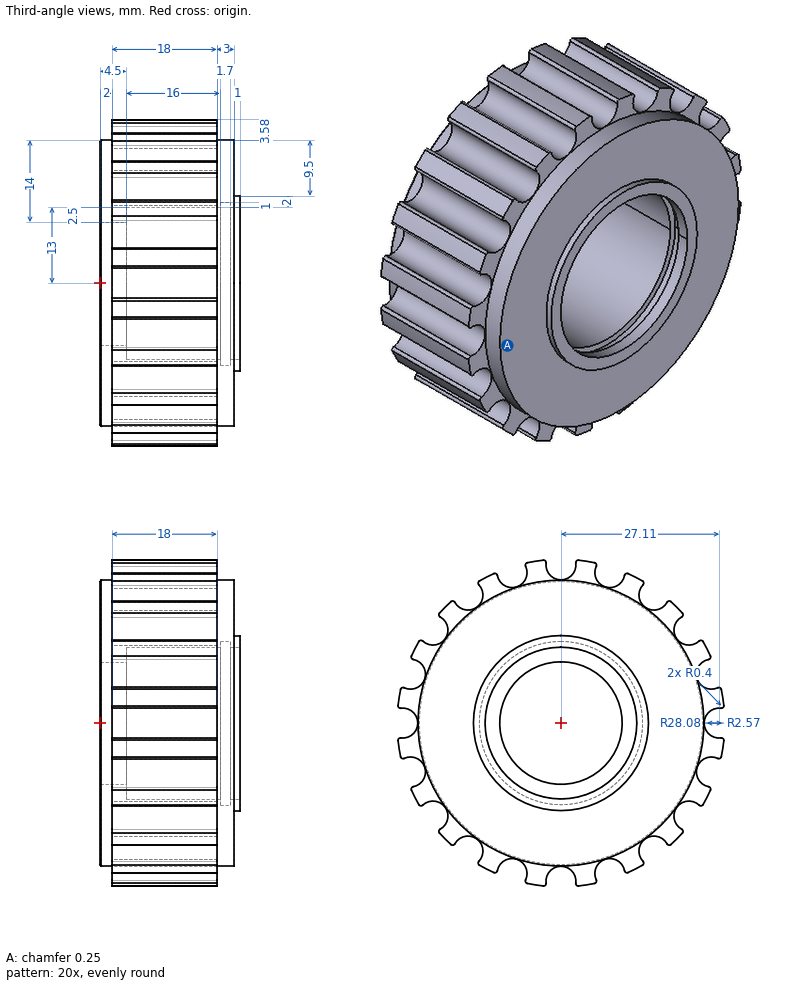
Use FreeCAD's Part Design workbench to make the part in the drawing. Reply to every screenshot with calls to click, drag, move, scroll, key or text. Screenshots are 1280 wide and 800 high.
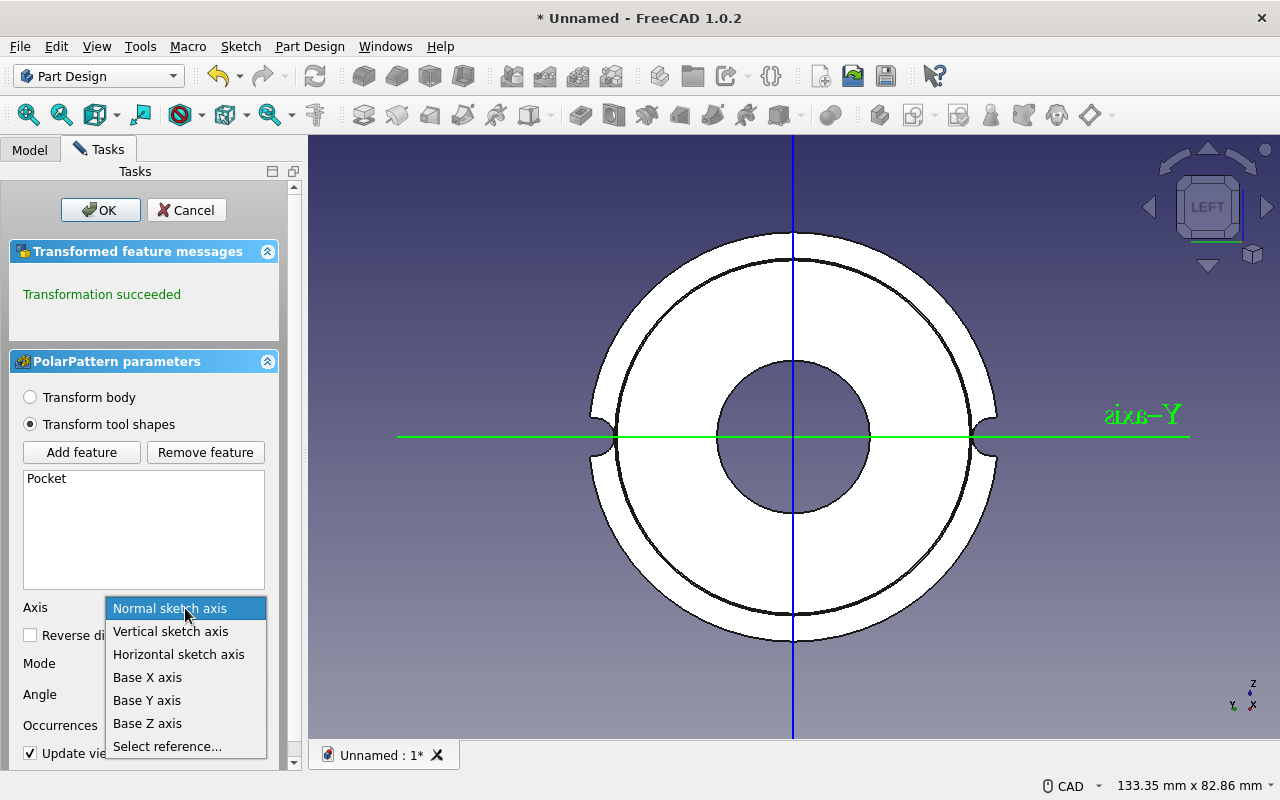
click(184, 678)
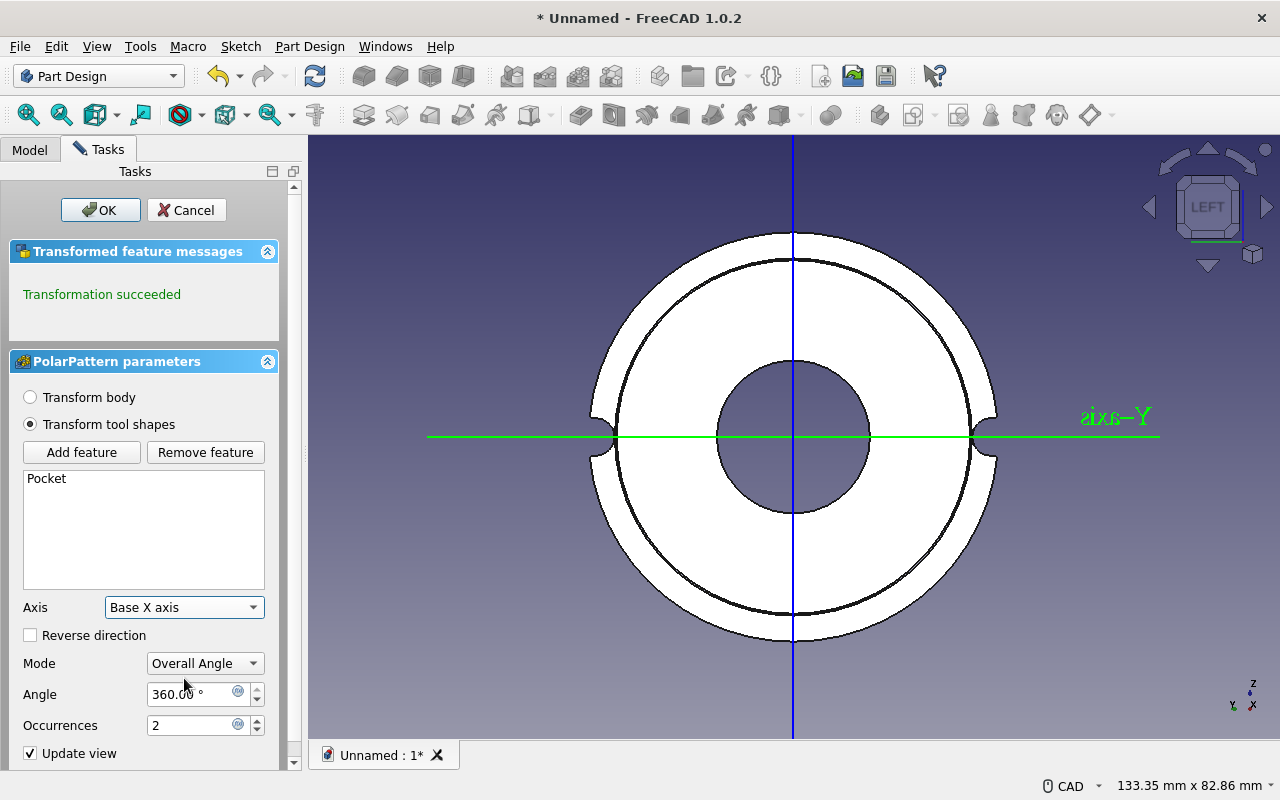
triple_click(199, 726)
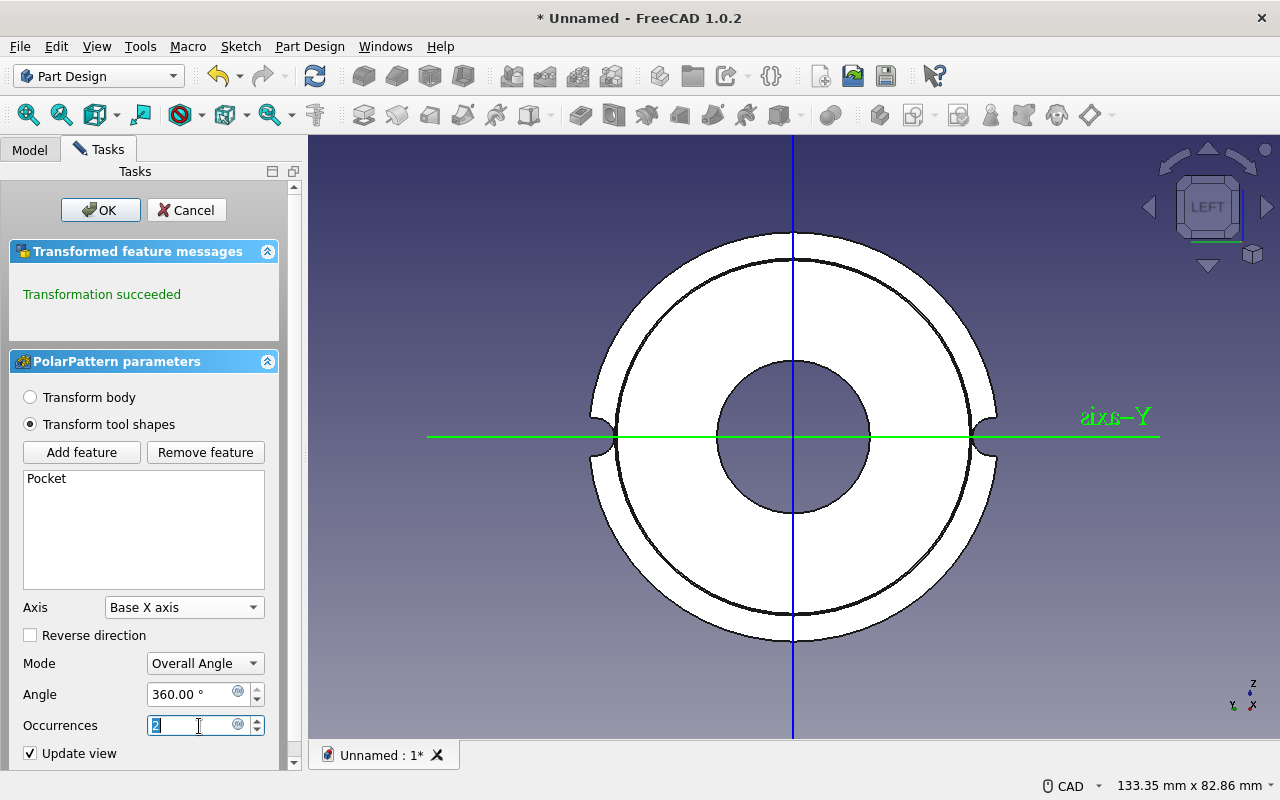
text(20)
key(Tab)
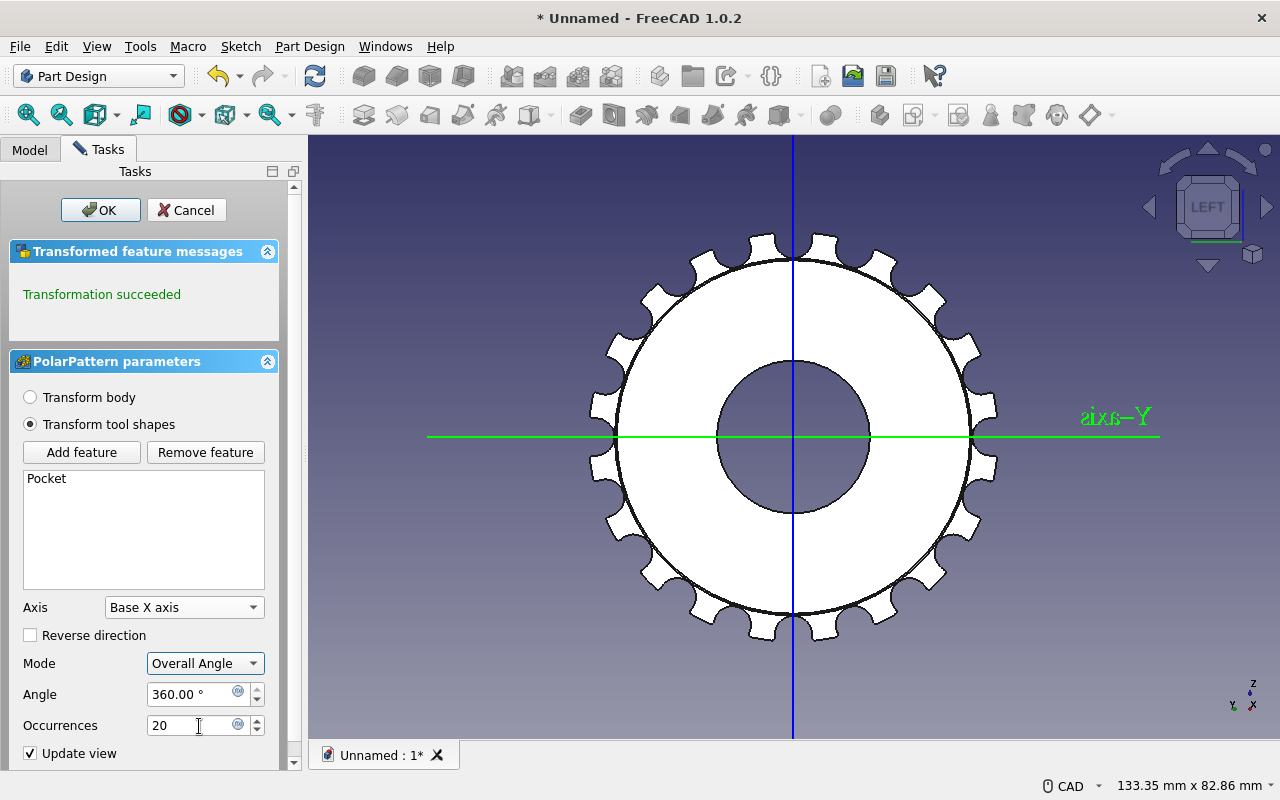
click(101, 210)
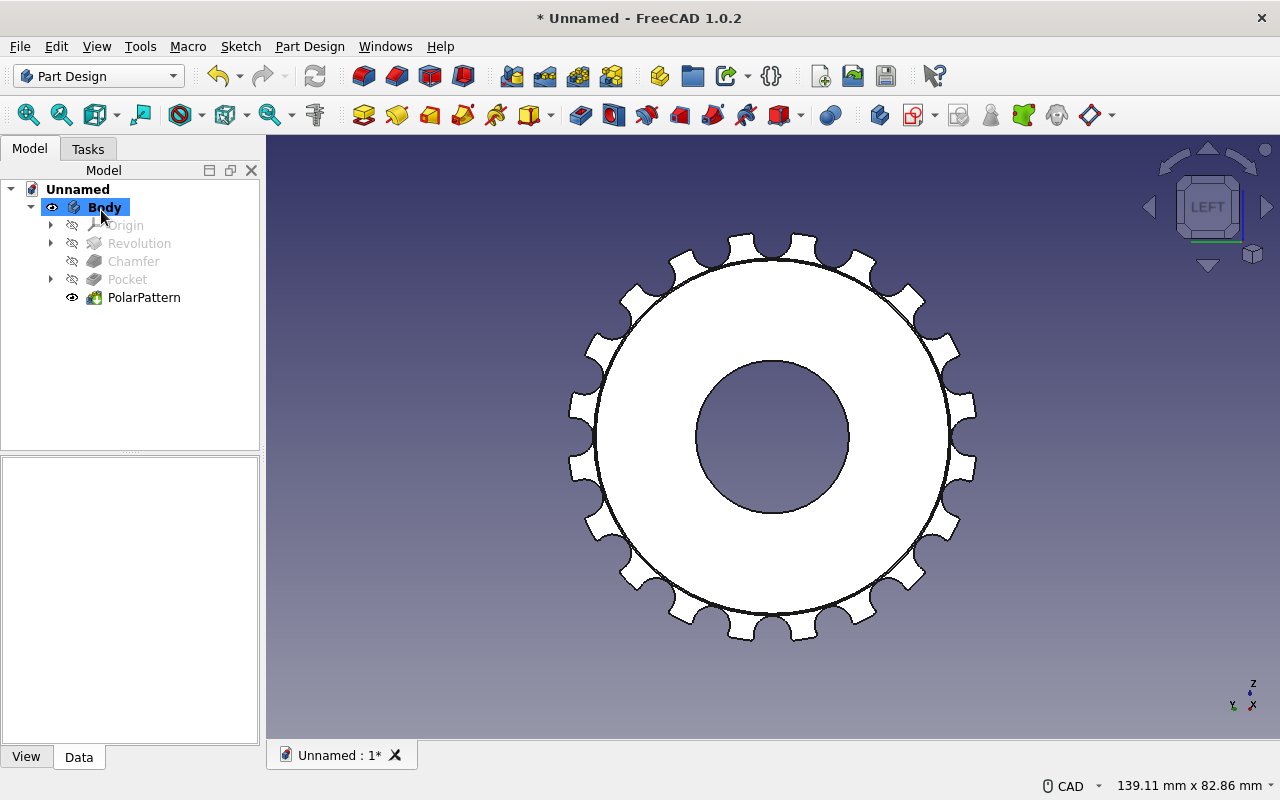
key(0)